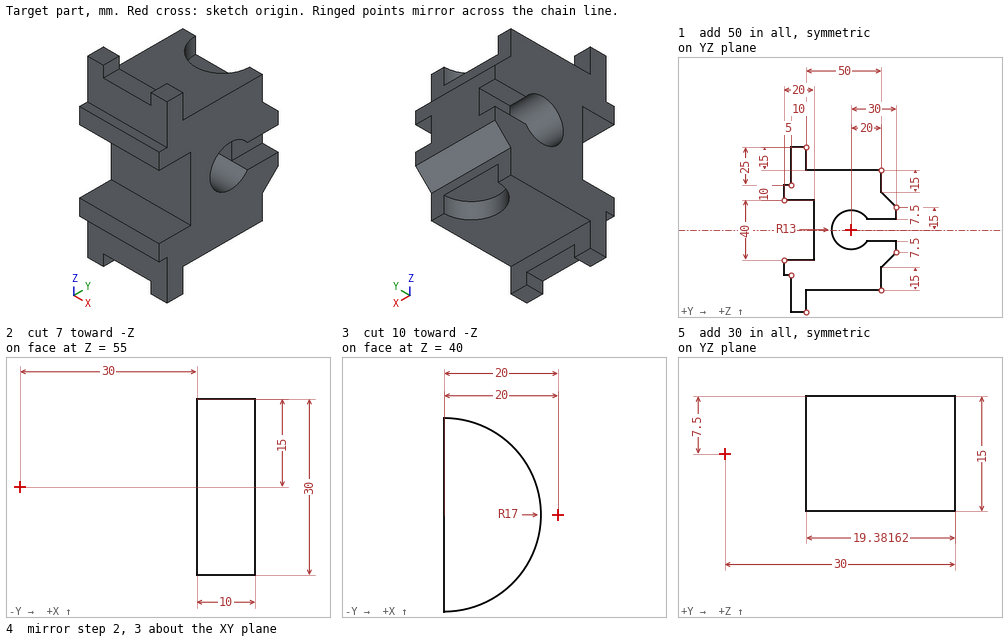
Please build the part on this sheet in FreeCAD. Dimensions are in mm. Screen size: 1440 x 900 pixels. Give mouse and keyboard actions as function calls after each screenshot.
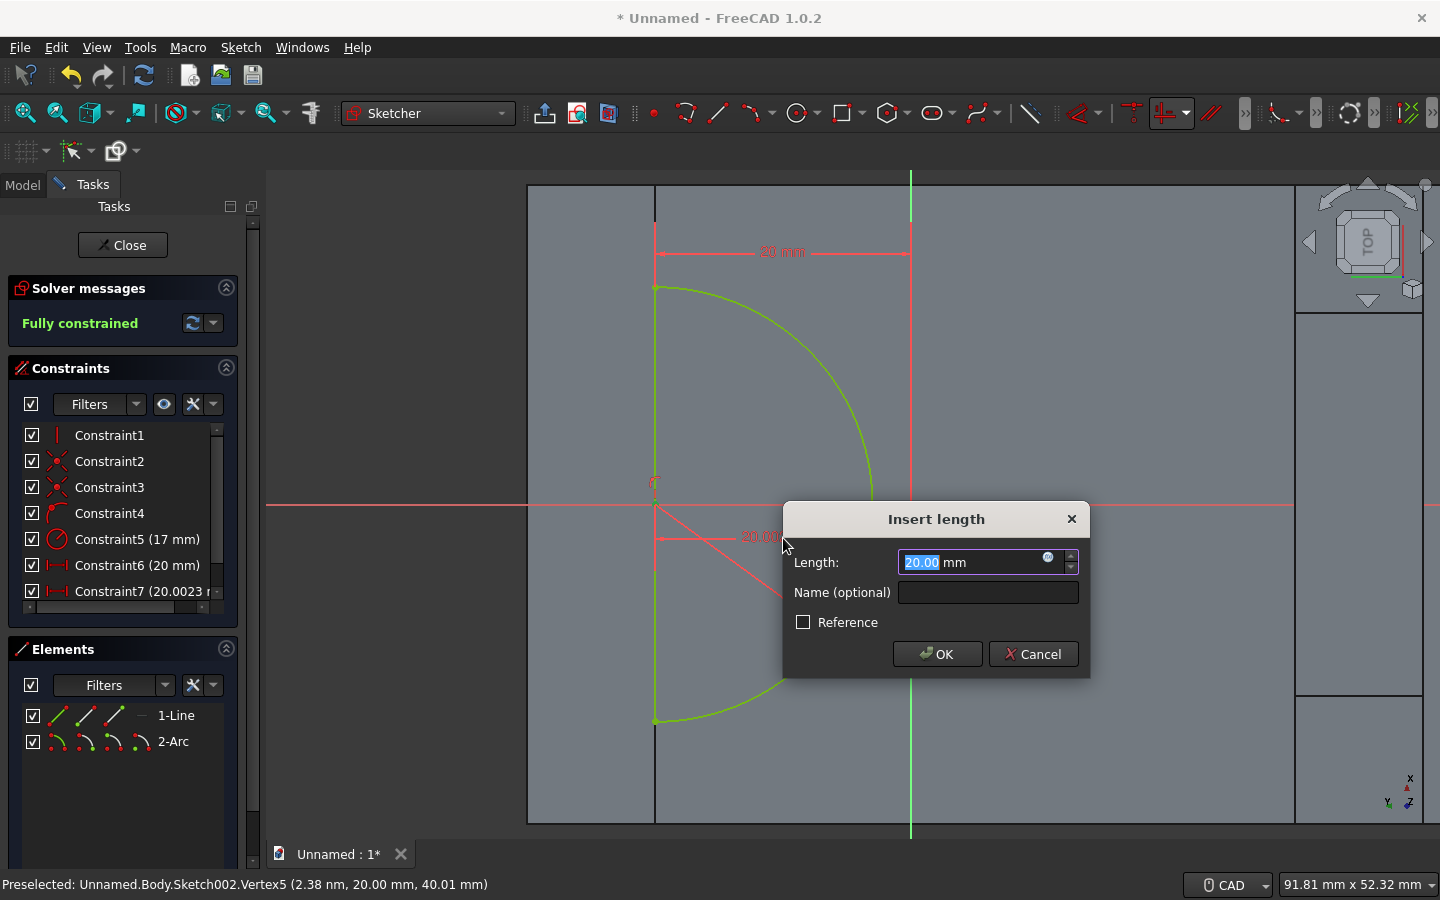
text(20)
key(Return)
key(Escape)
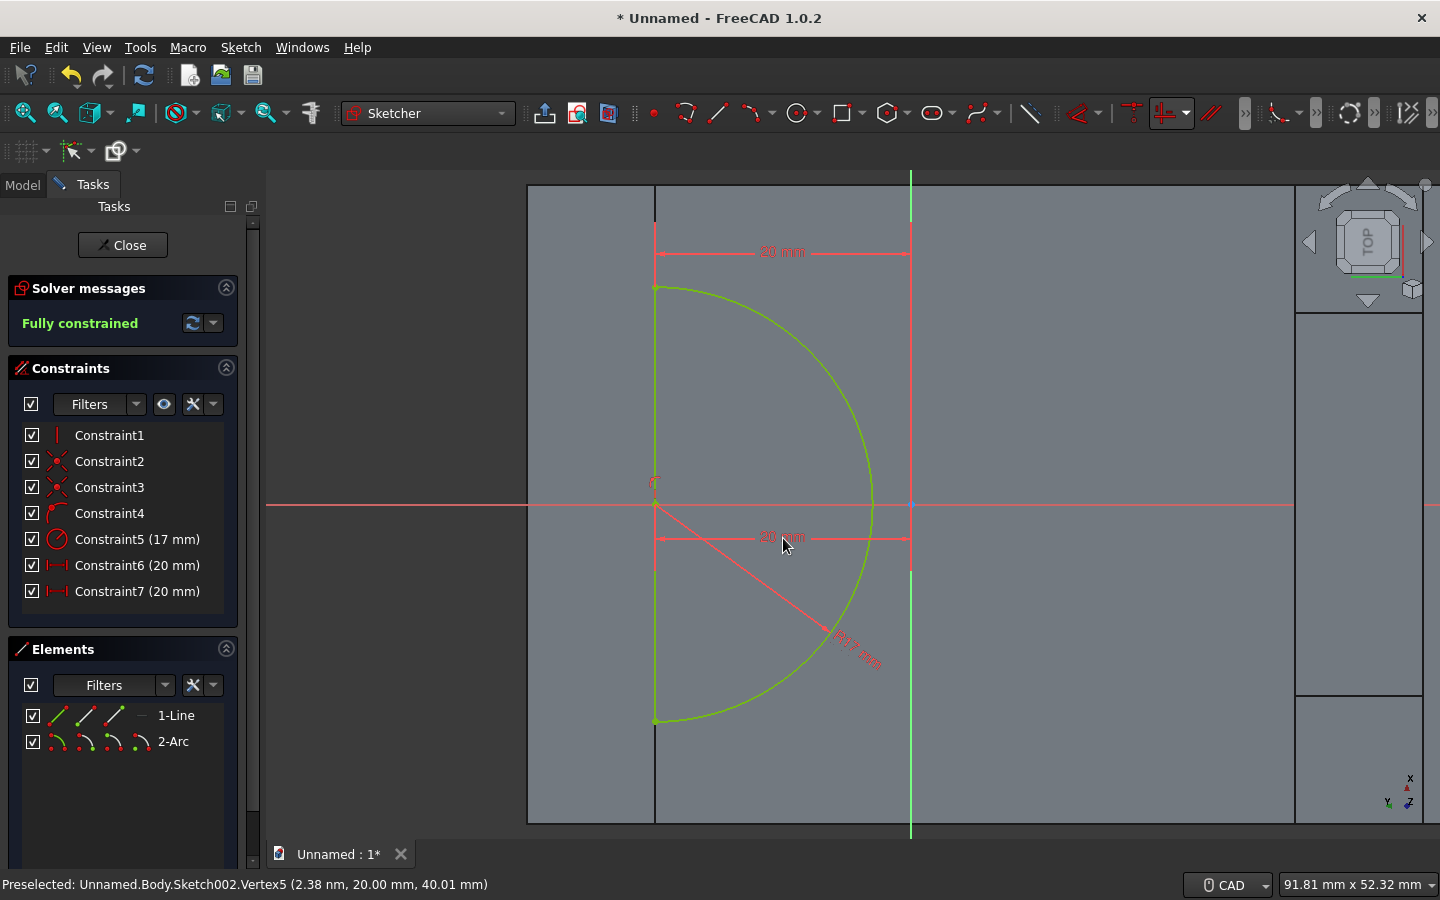
click(123, 245)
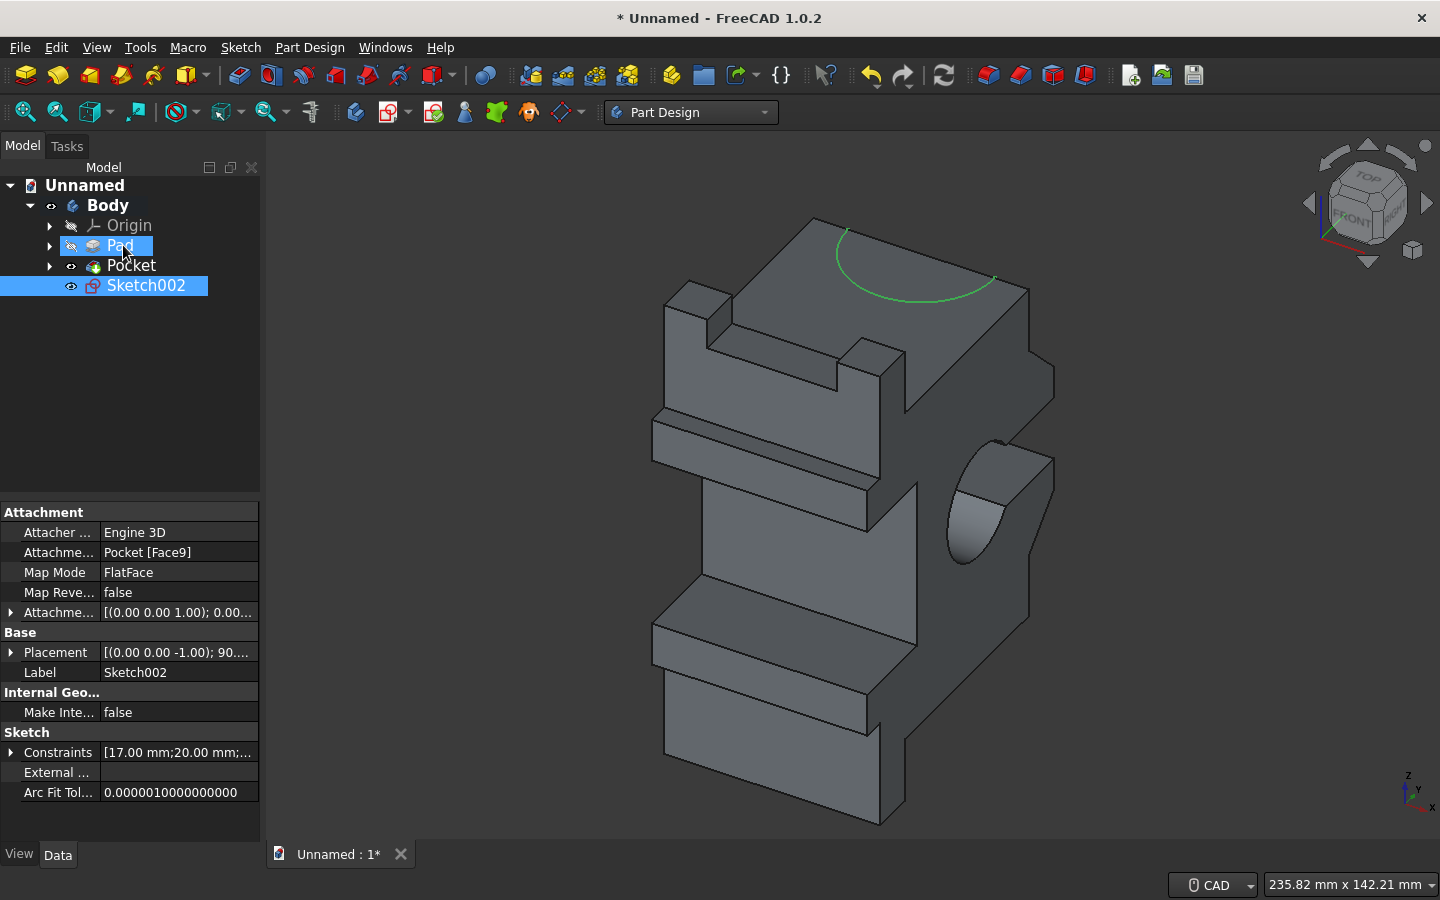
click(240, 76)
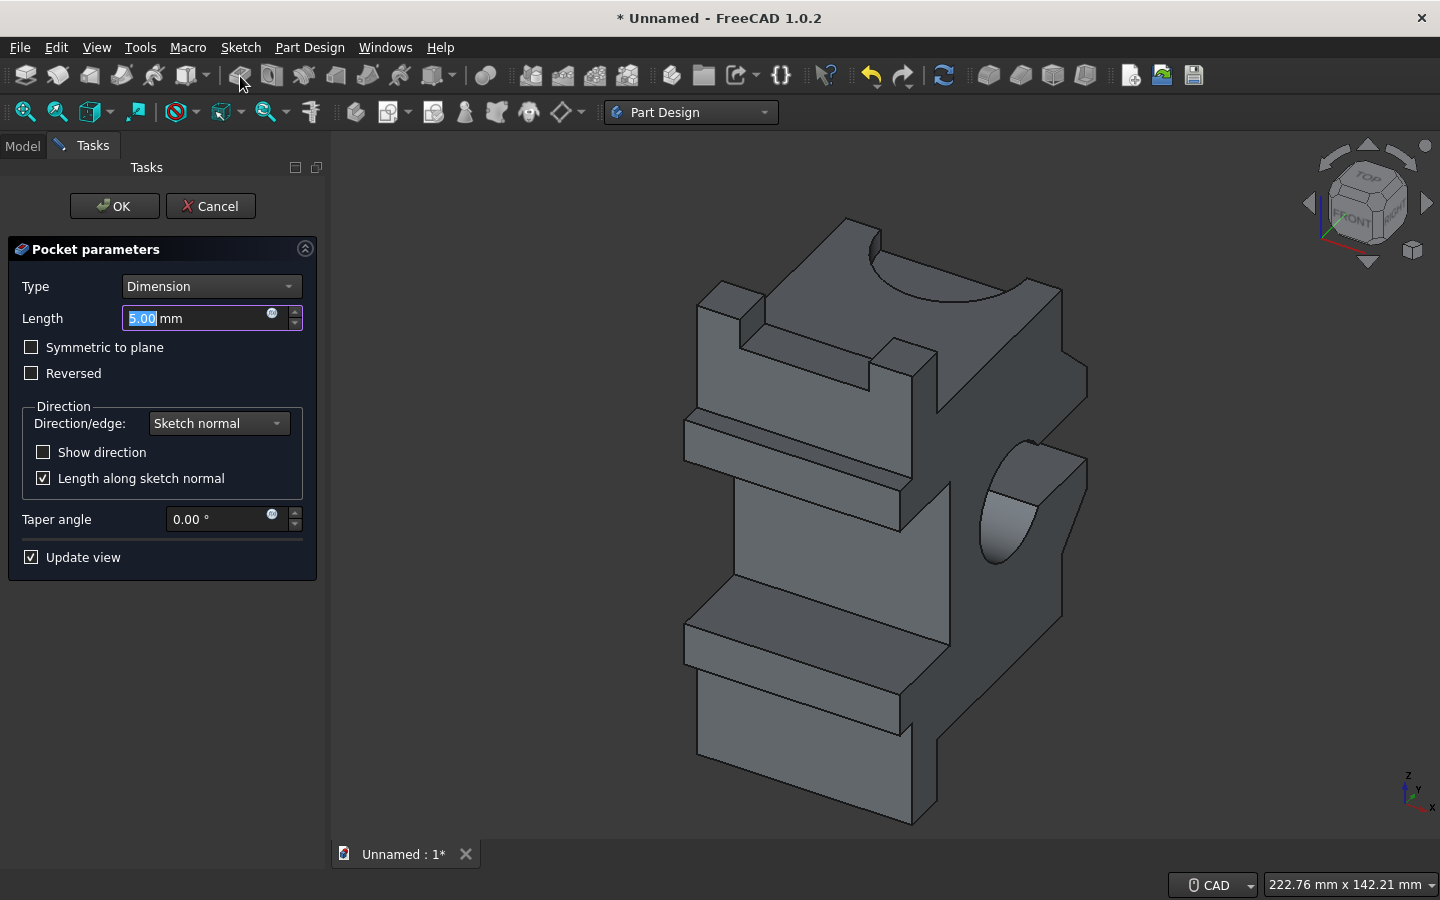
text(10)
key(Tab)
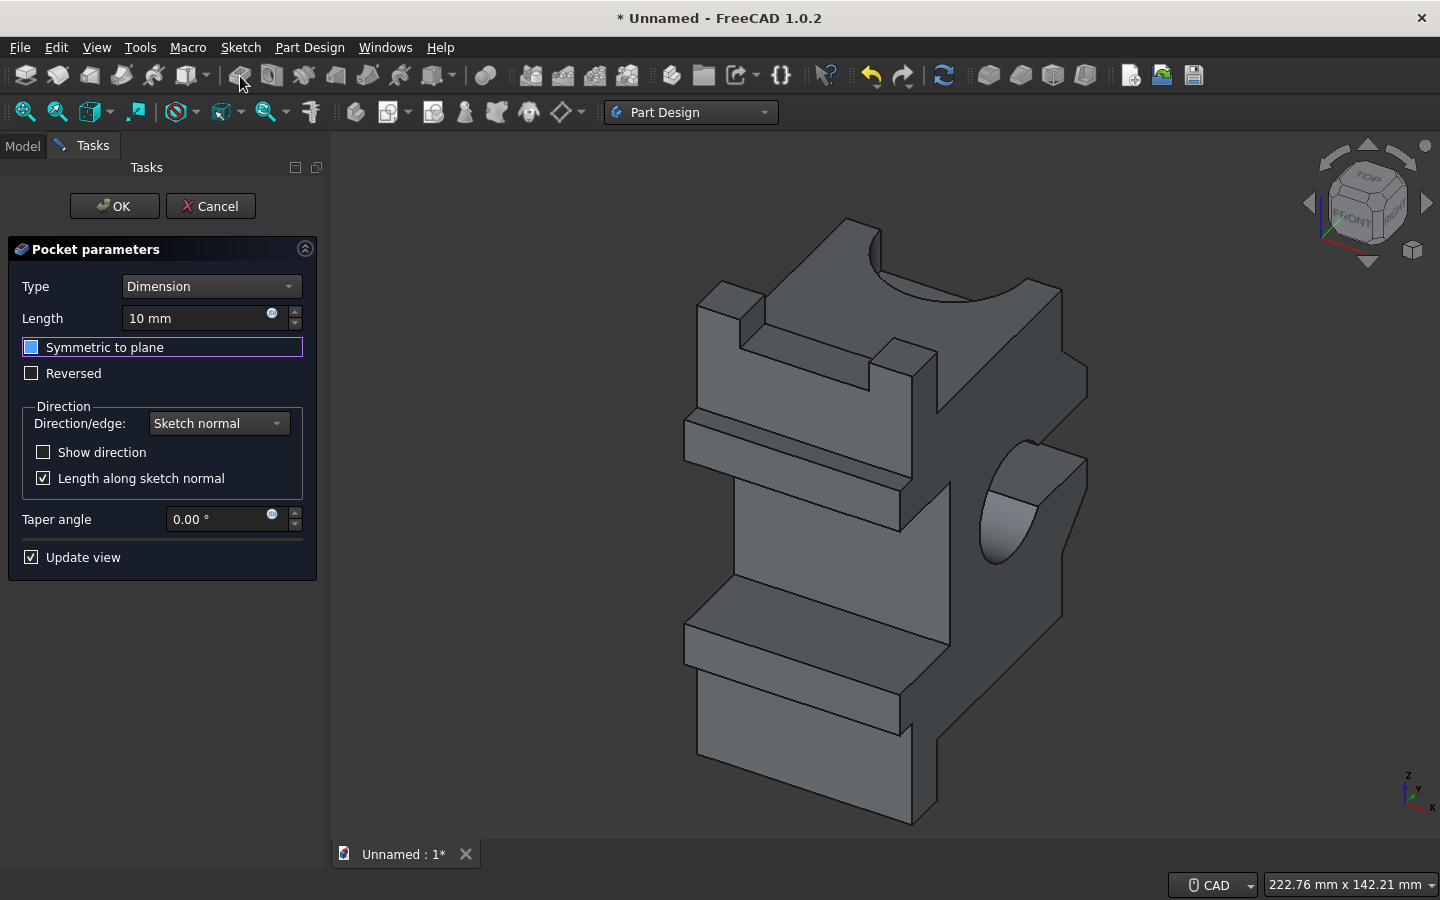
click(115, 206)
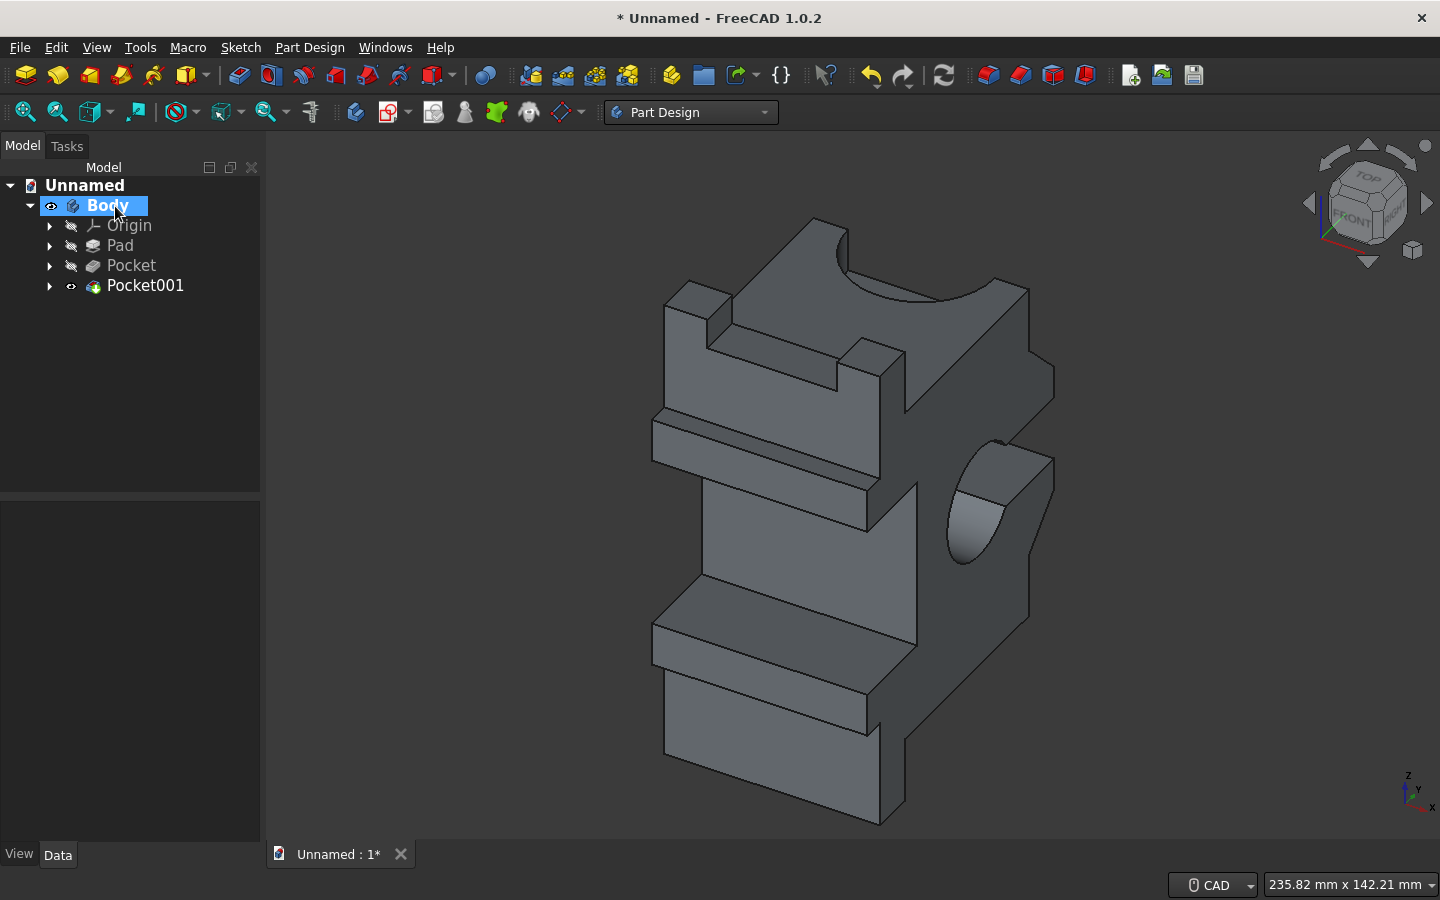
click(116, 266)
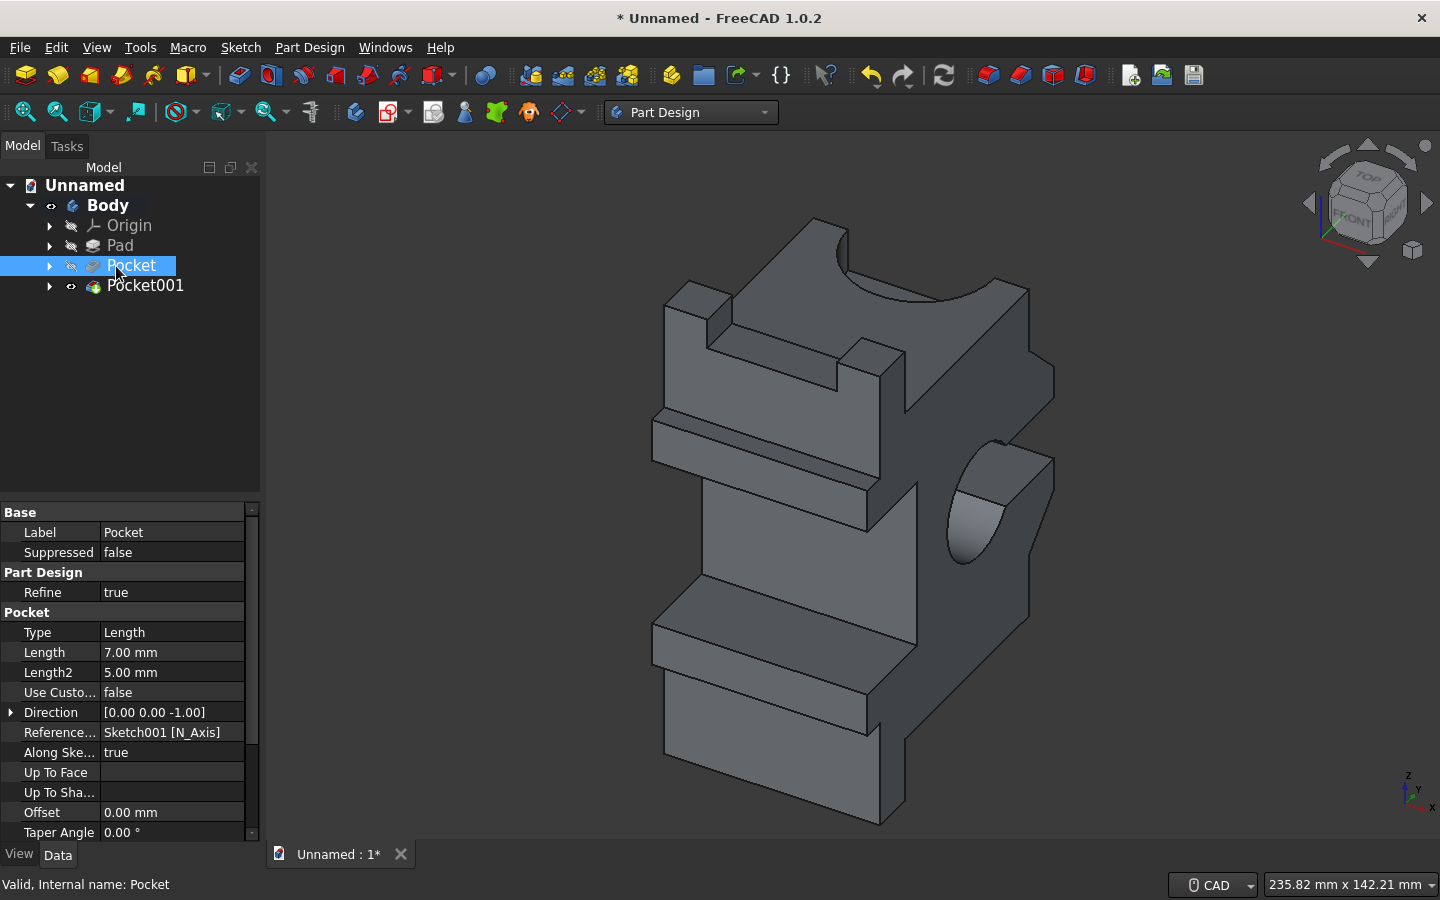
click(116, 286, ctrl)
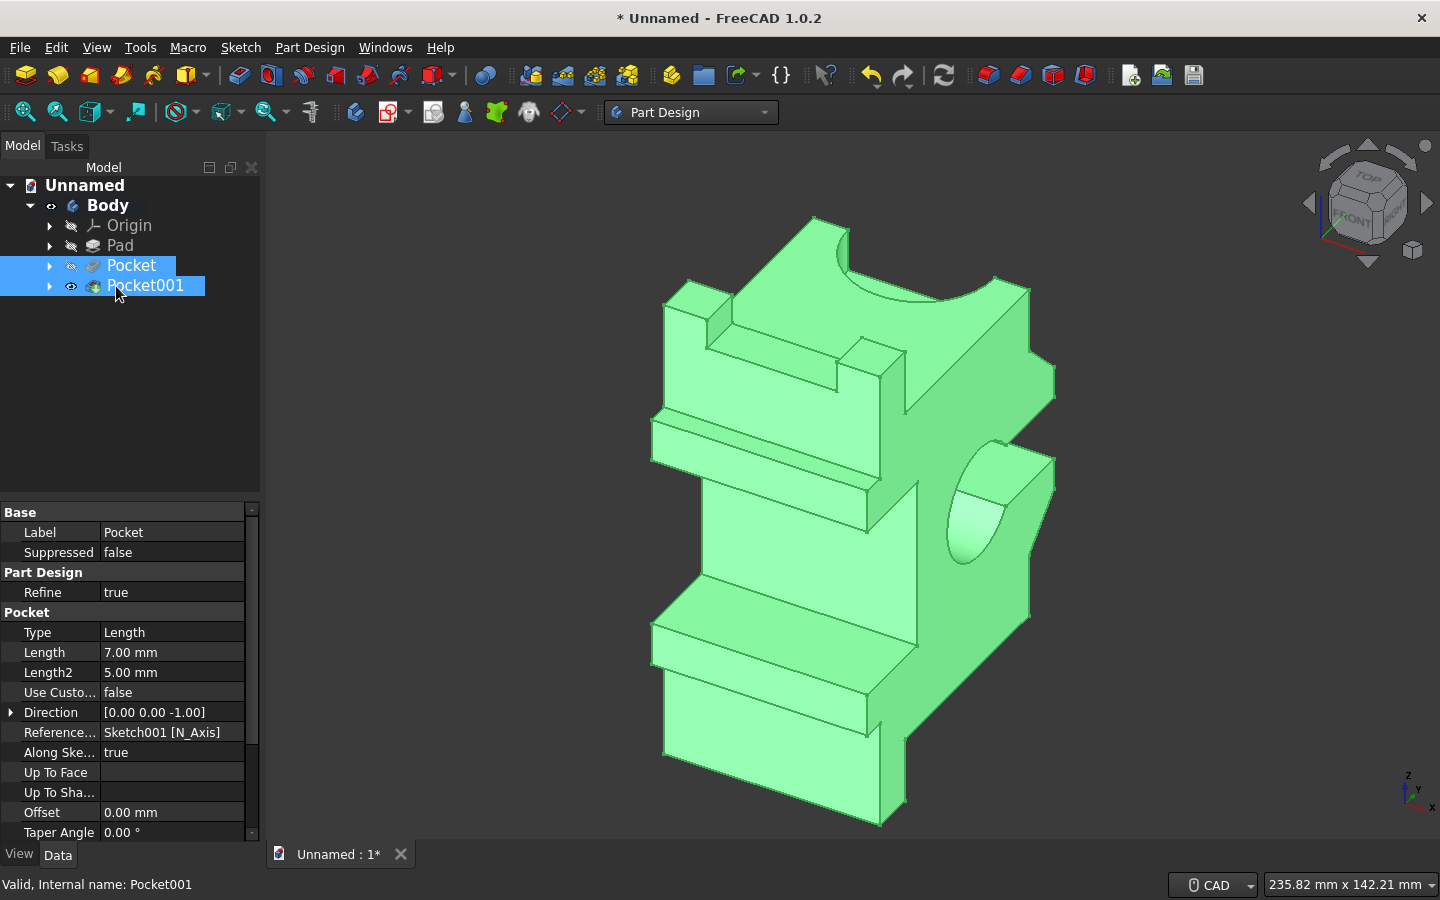
click(532, 76)